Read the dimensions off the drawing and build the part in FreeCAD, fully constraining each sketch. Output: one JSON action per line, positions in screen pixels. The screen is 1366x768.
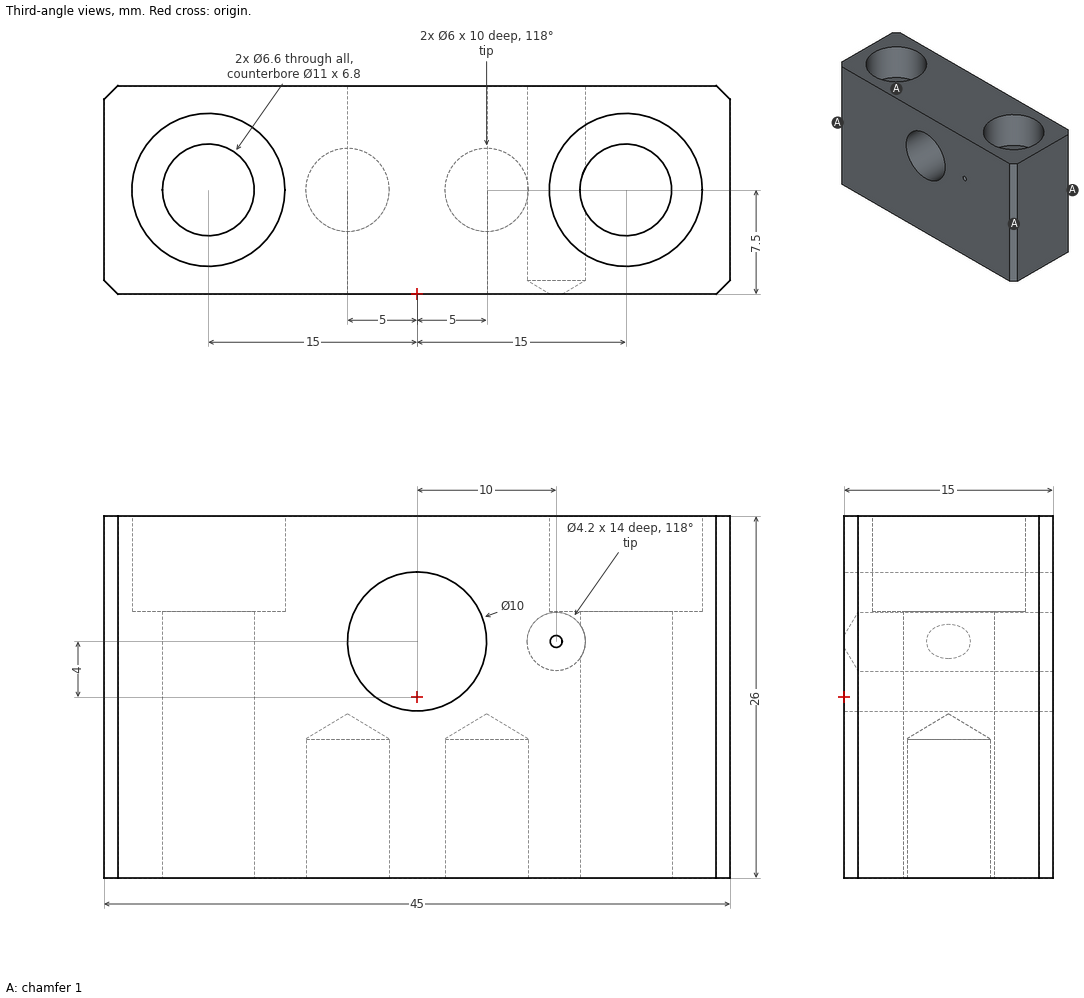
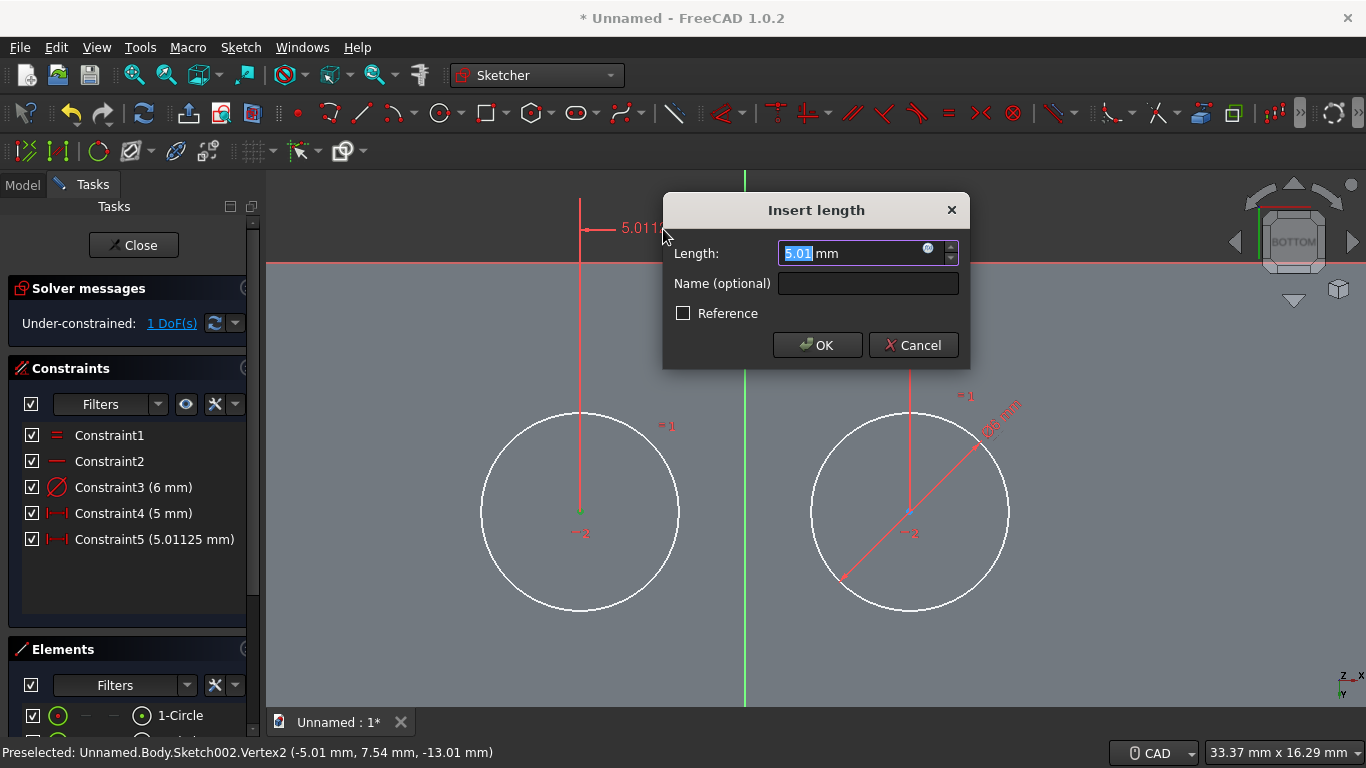
{"action": "type", "text": "5"}
{"action": "key", "text": "Return"}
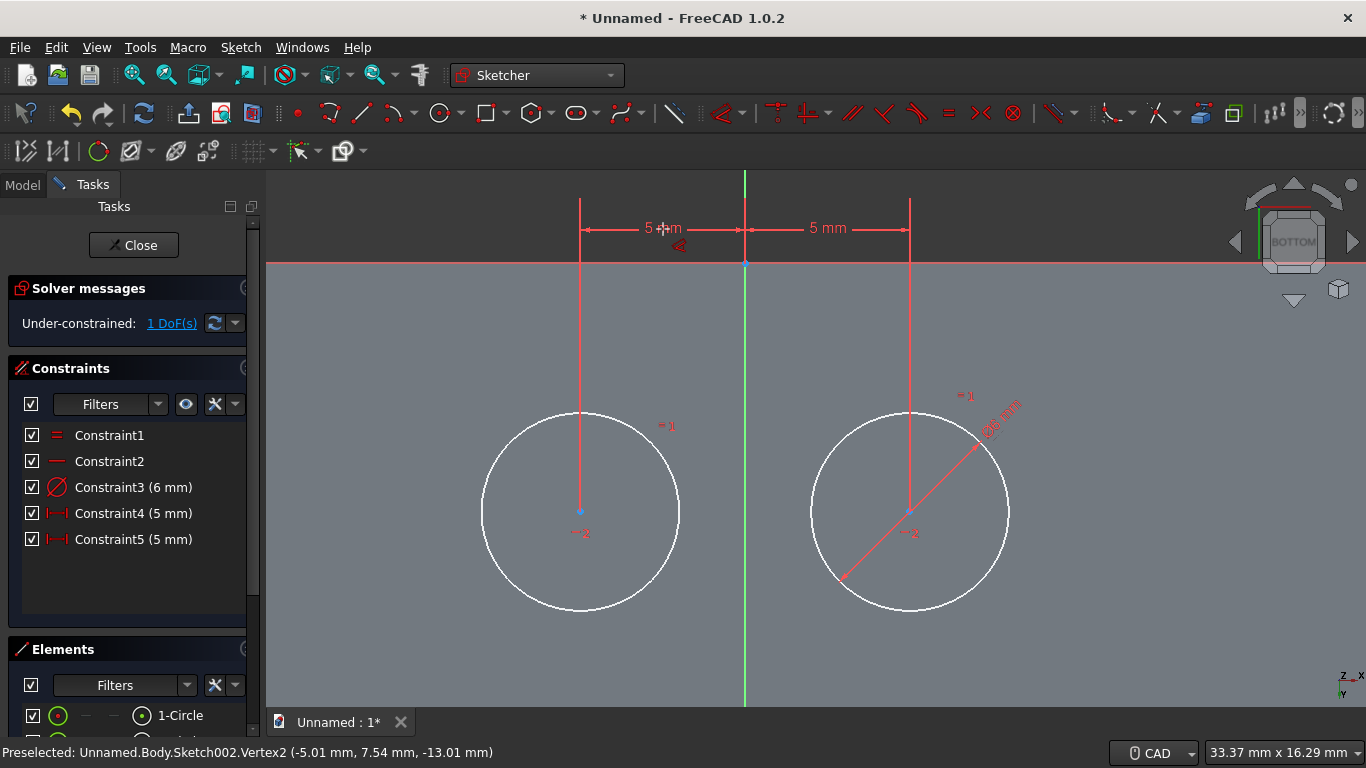
{"action": "left_click", "coordinate": [910, 512]}
{"action": "left_click", "coordinate": [944, 388]}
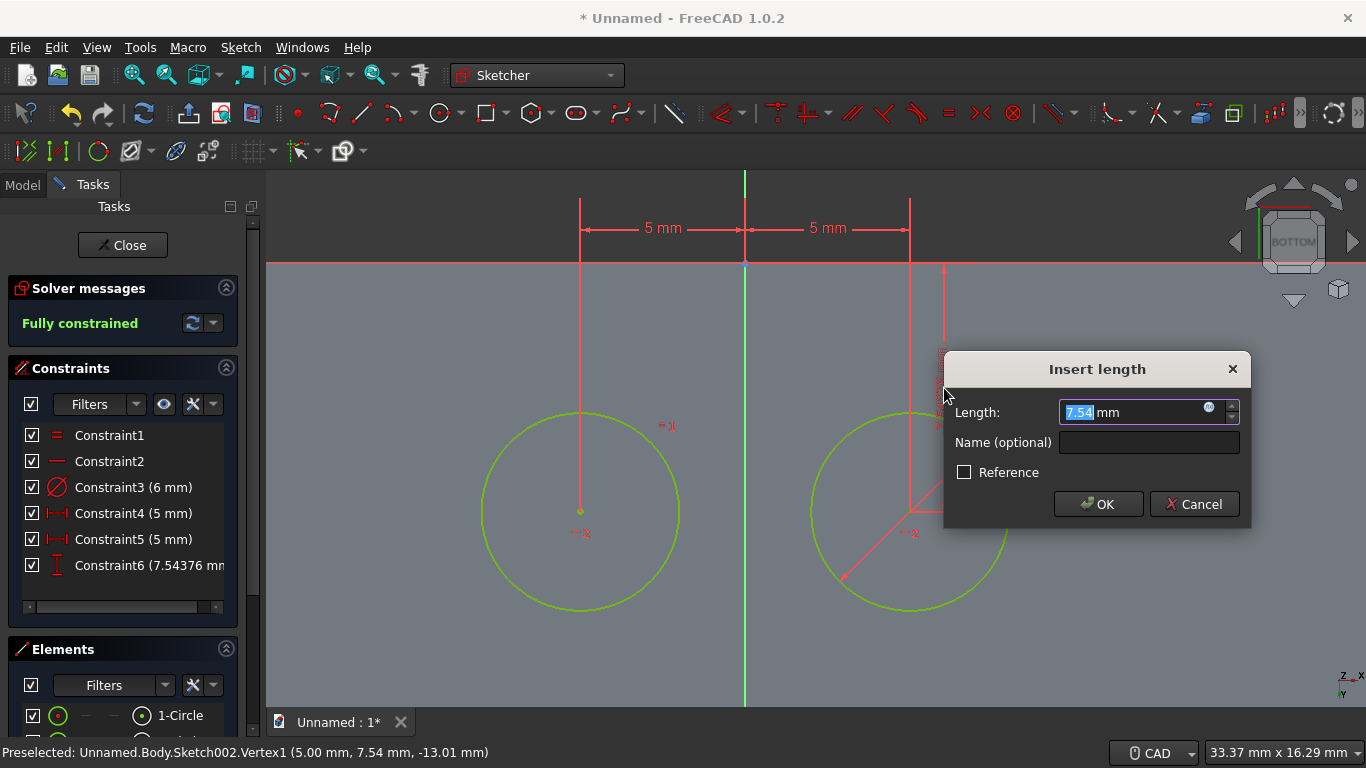
{"action": "type", "text": "7.5"}
{"action": "key", "text": "Return"}
{"action": "key", "text": "Escape"}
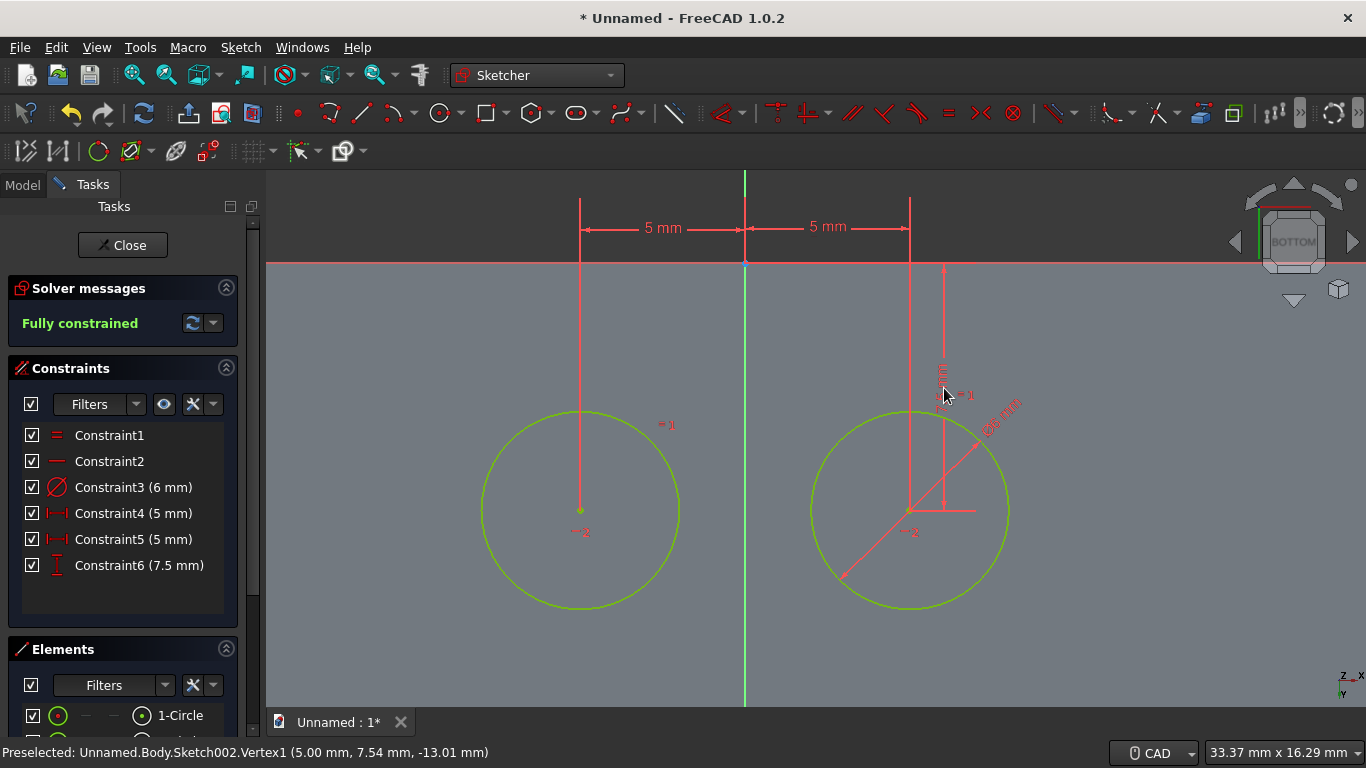
{"action": "left_click", "coordinate": [123, 245]}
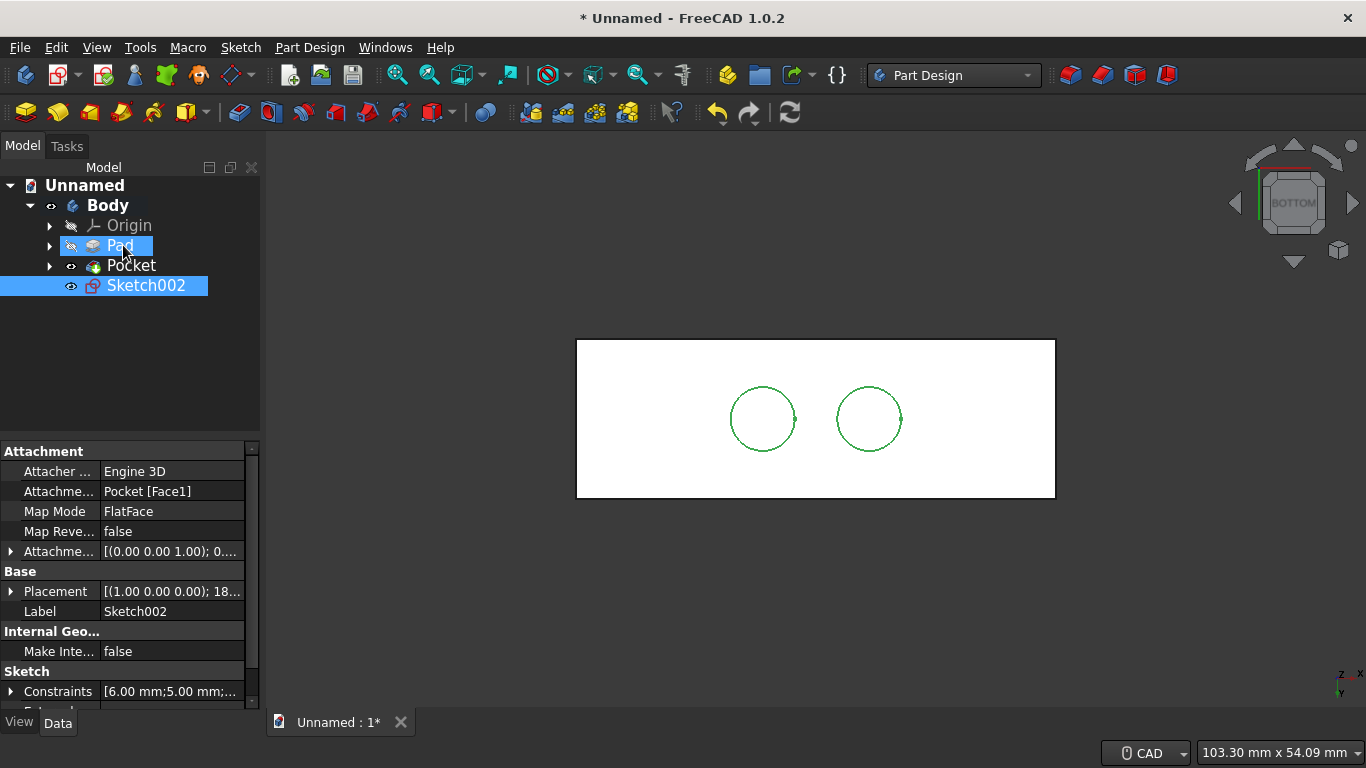
{"action": "left_click", "coordinate": [272, 112]}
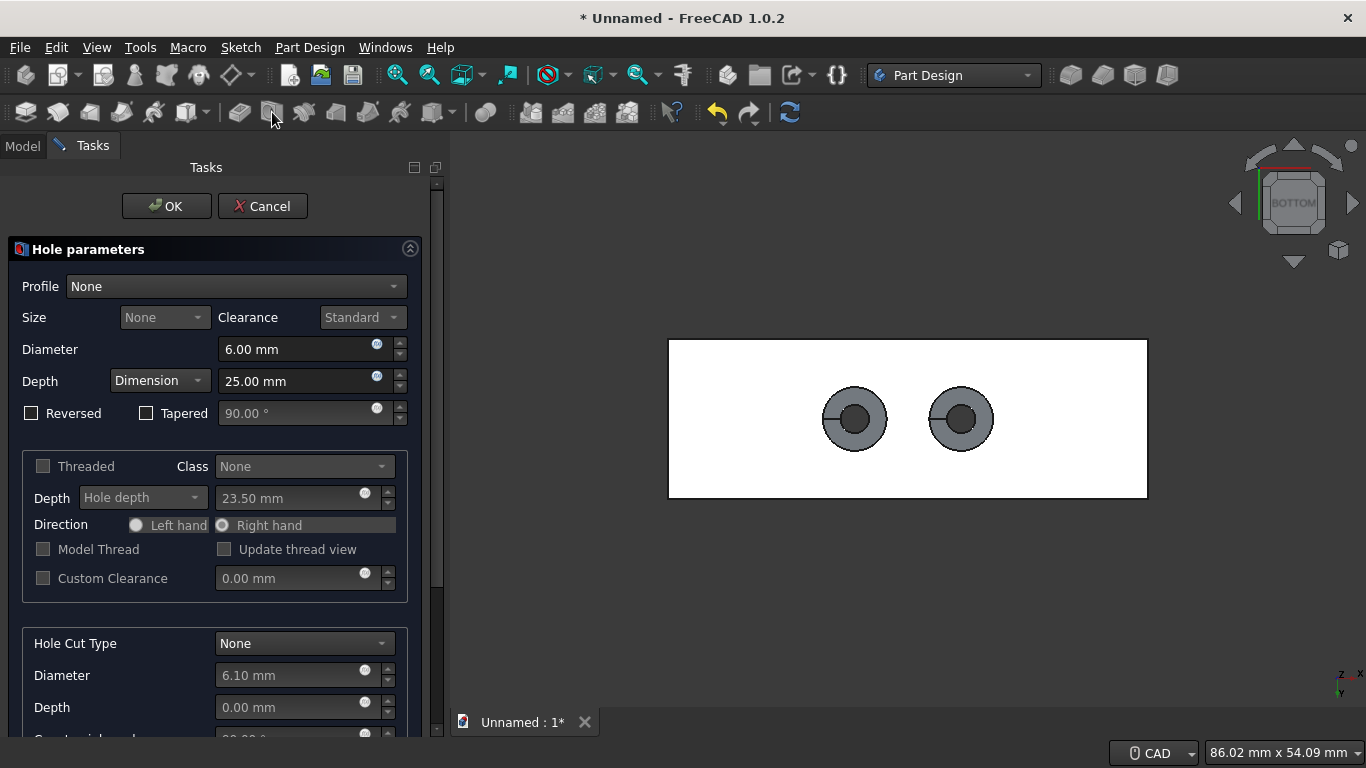
{"action": "triple_click", "coordinate": [305, 349]}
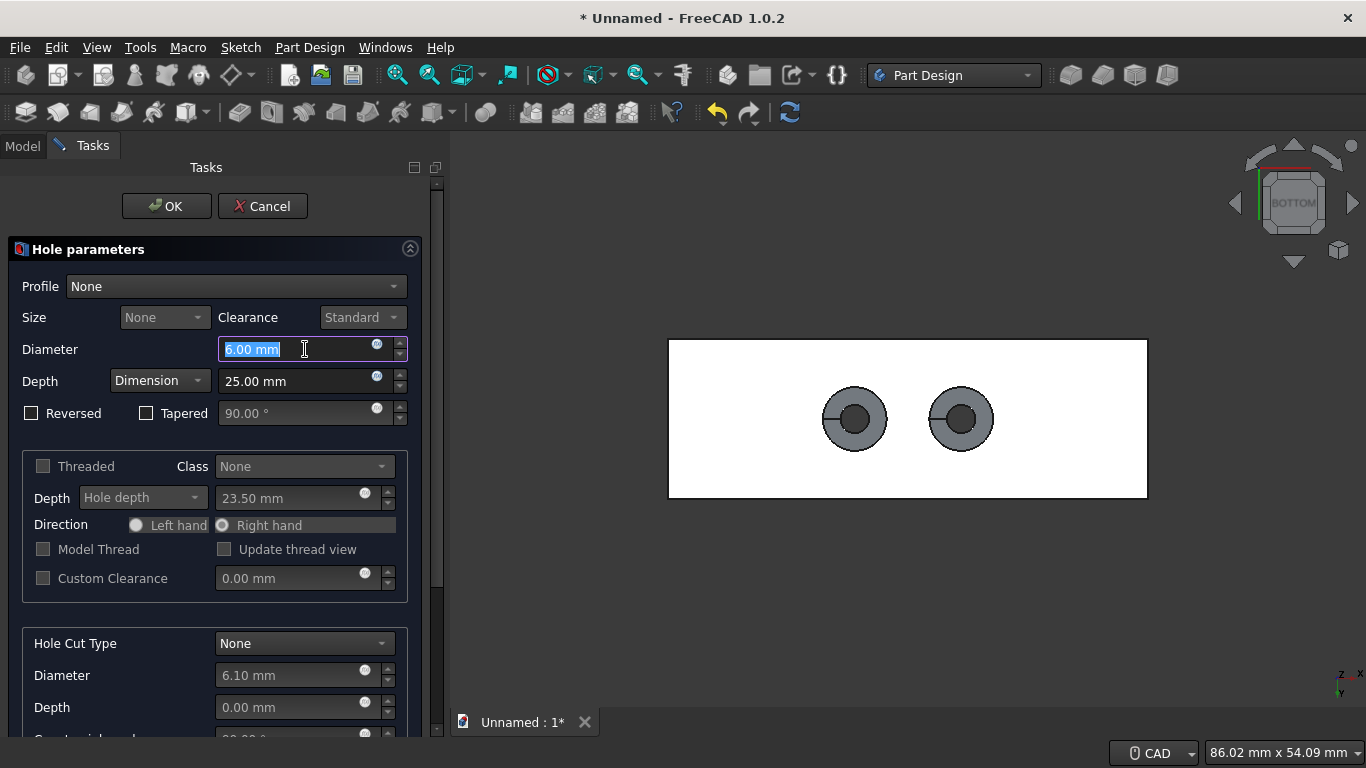
{"action": "type", "text": "6"}
{"action": "key", "text": "Tab"}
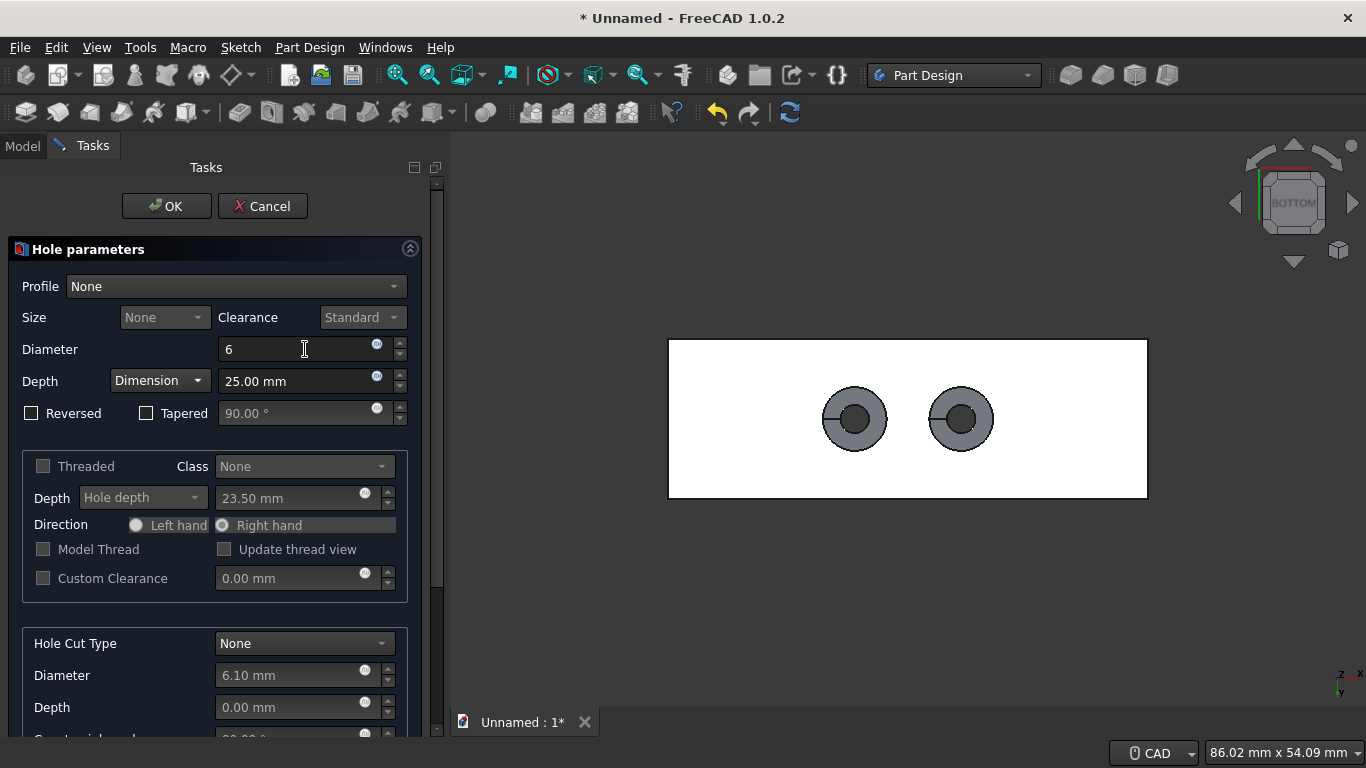
{"action": "triple_click", "coordinate": [305, 381]}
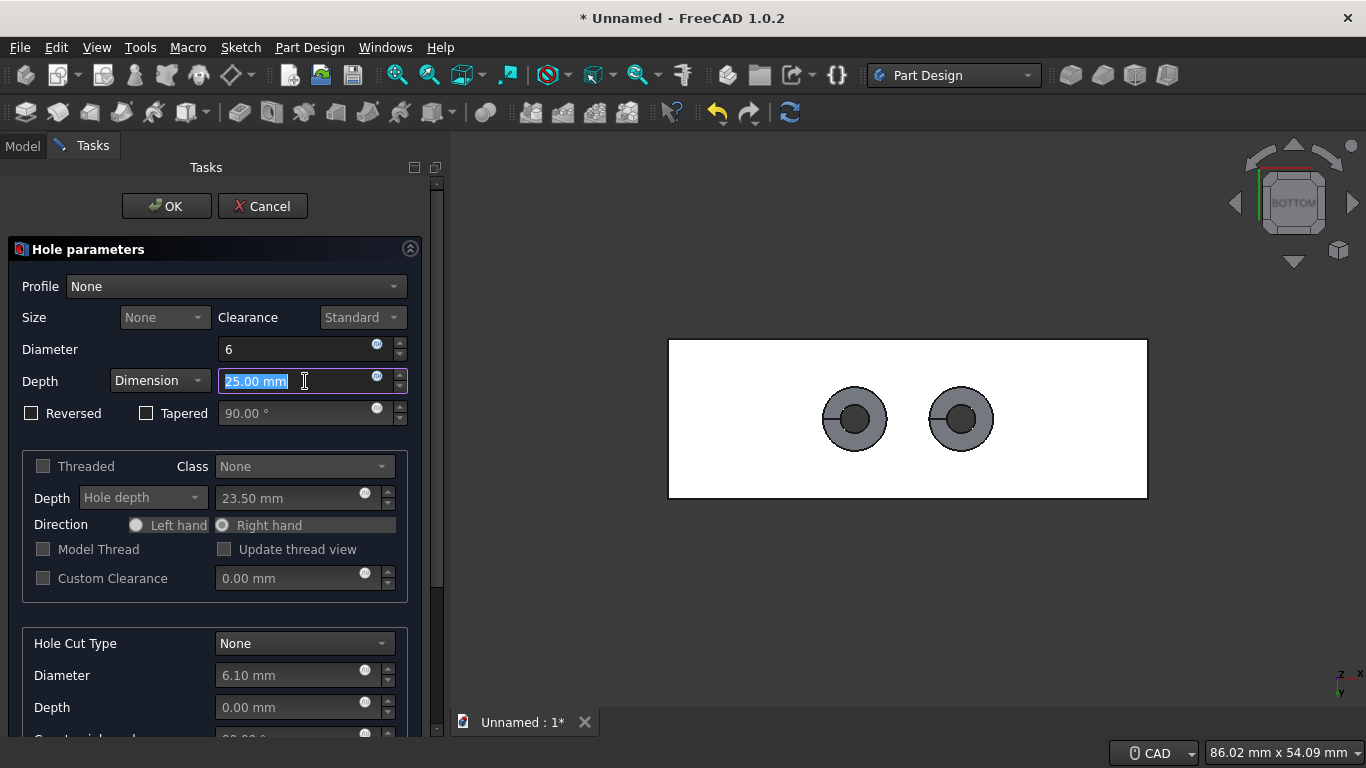
{"action": "type", "text": "10"}
{"action": "key", "text": "Tab"}